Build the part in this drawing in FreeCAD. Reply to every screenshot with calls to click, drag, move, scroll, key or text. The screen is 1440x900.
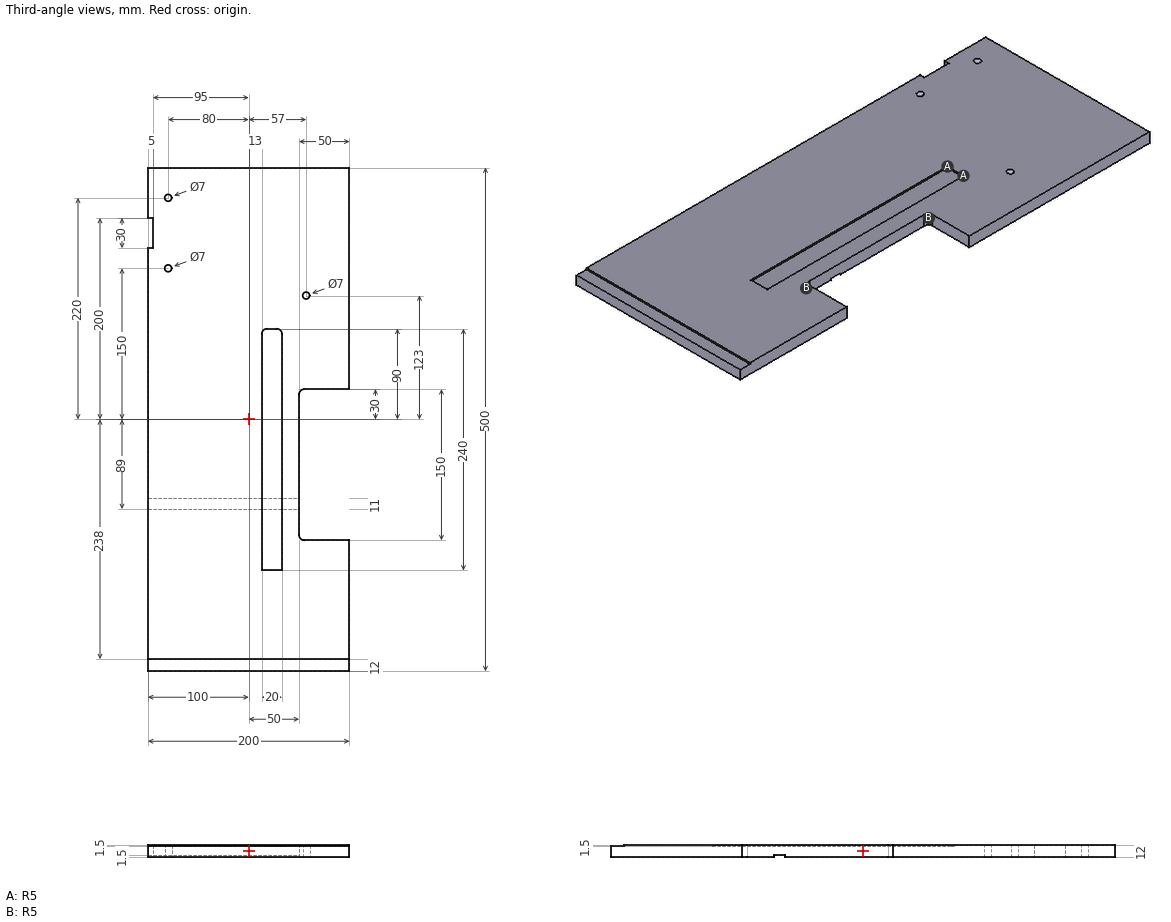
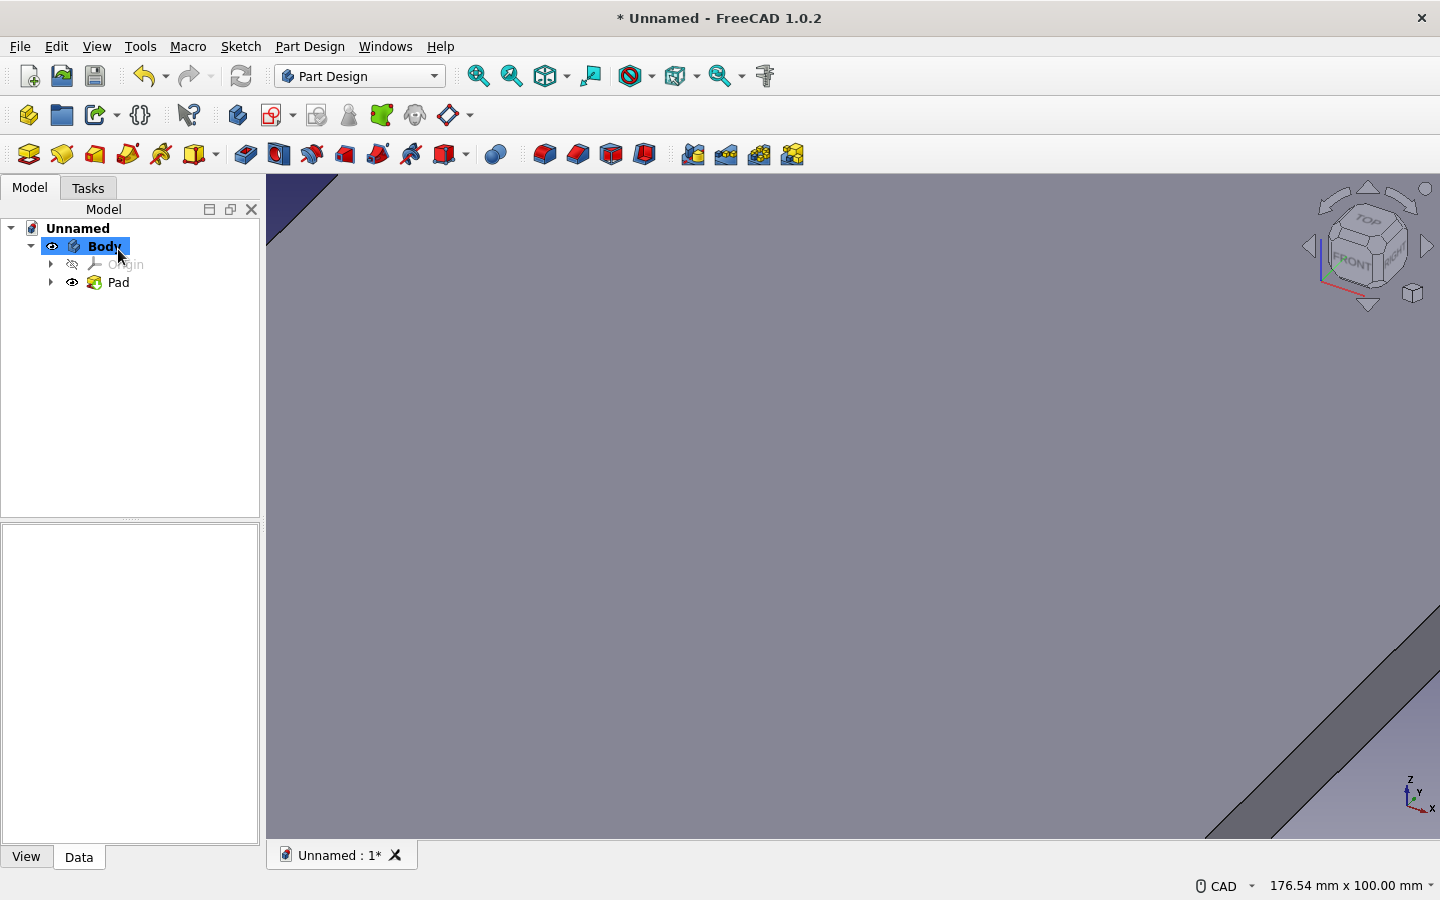
click(479, 76)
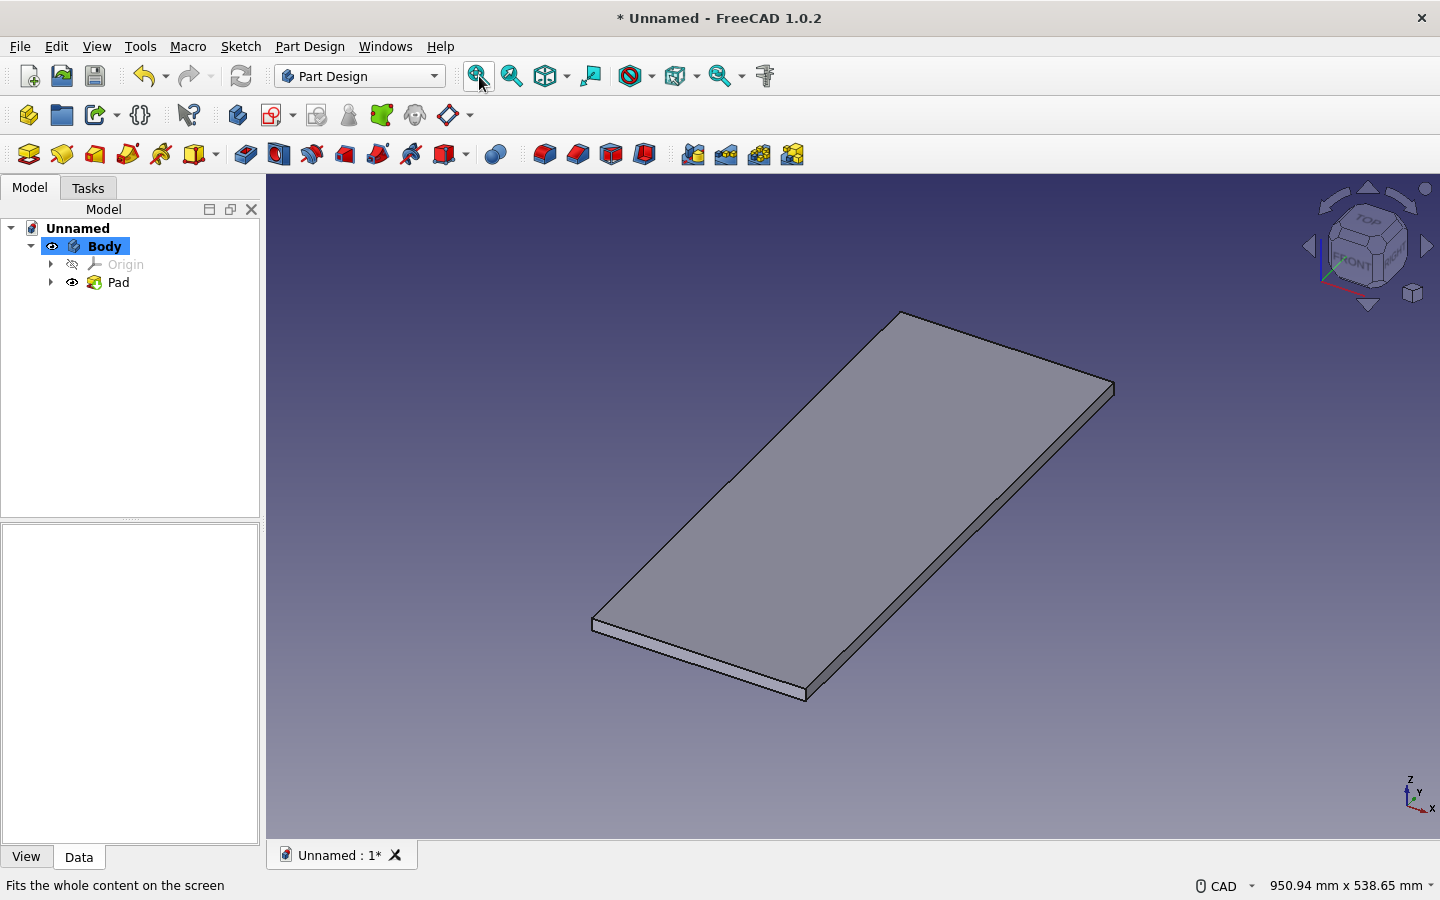
key(5)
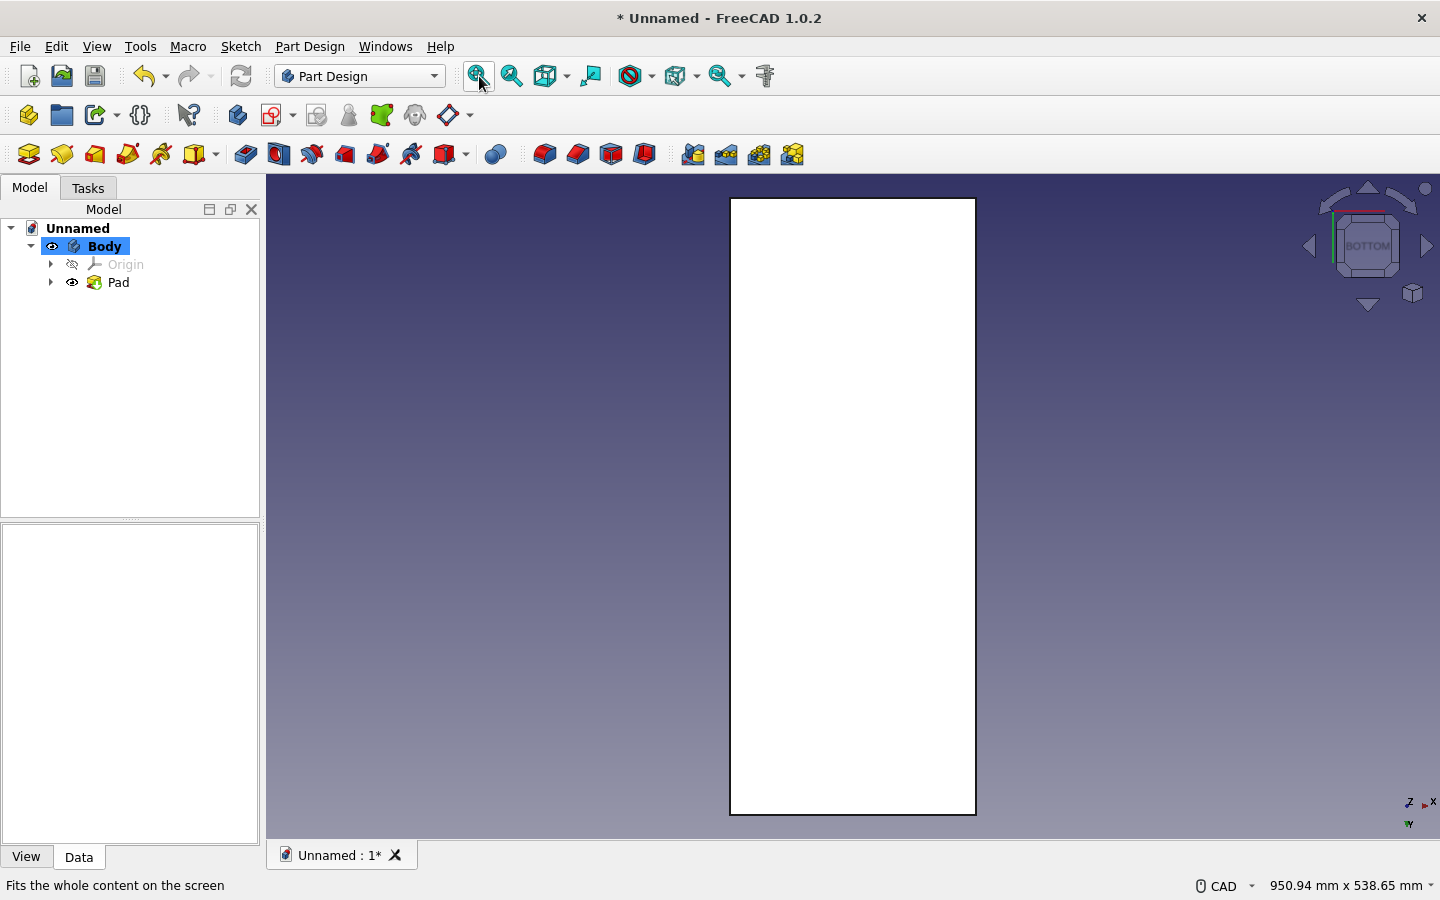
click(853, 682)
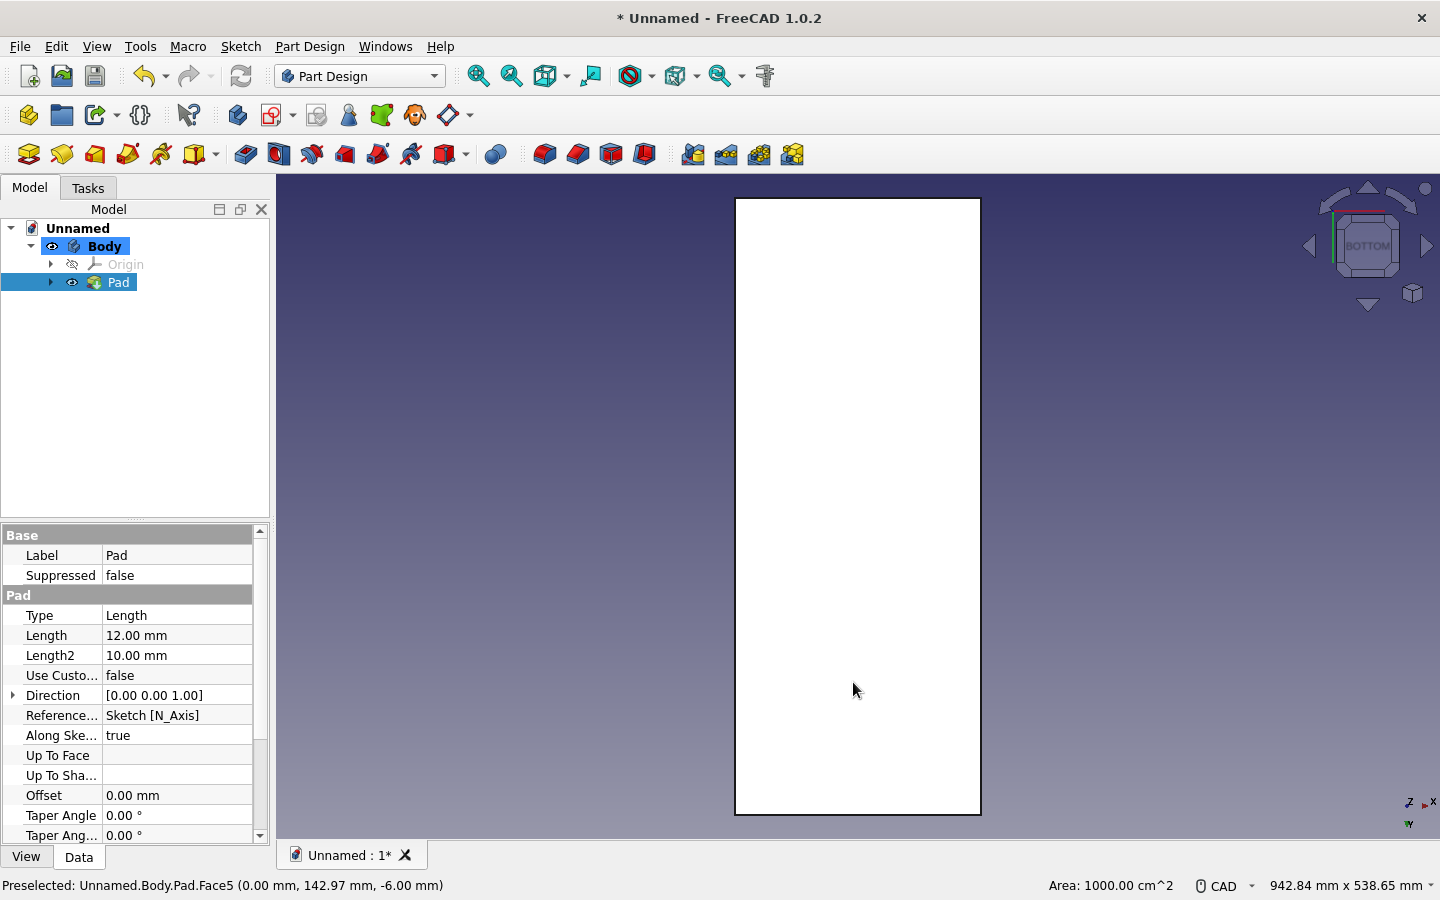
click(270, 116)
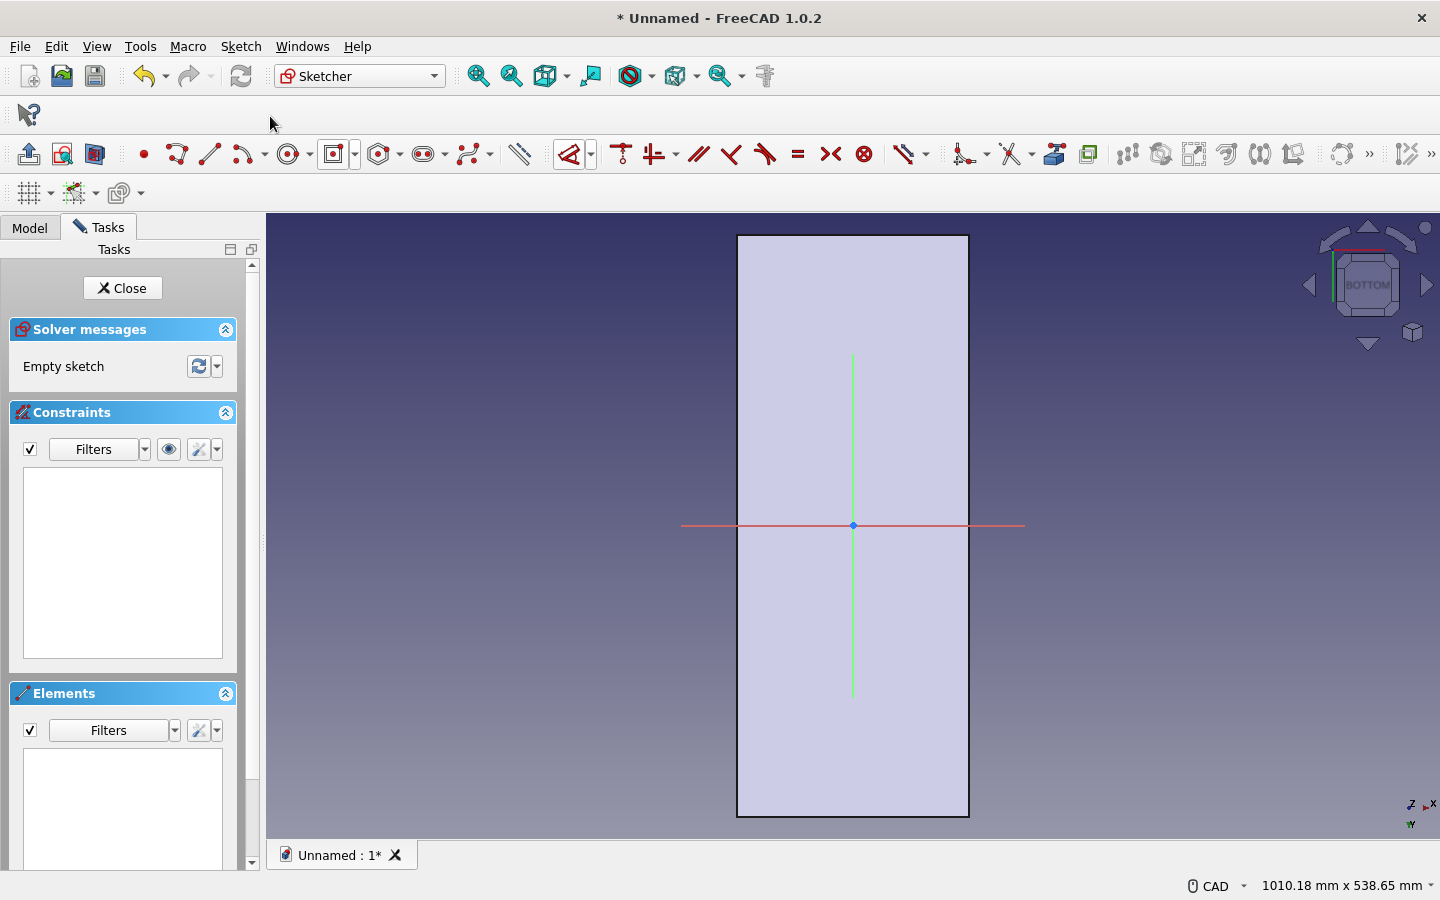
scroll(893, 444, up, 5)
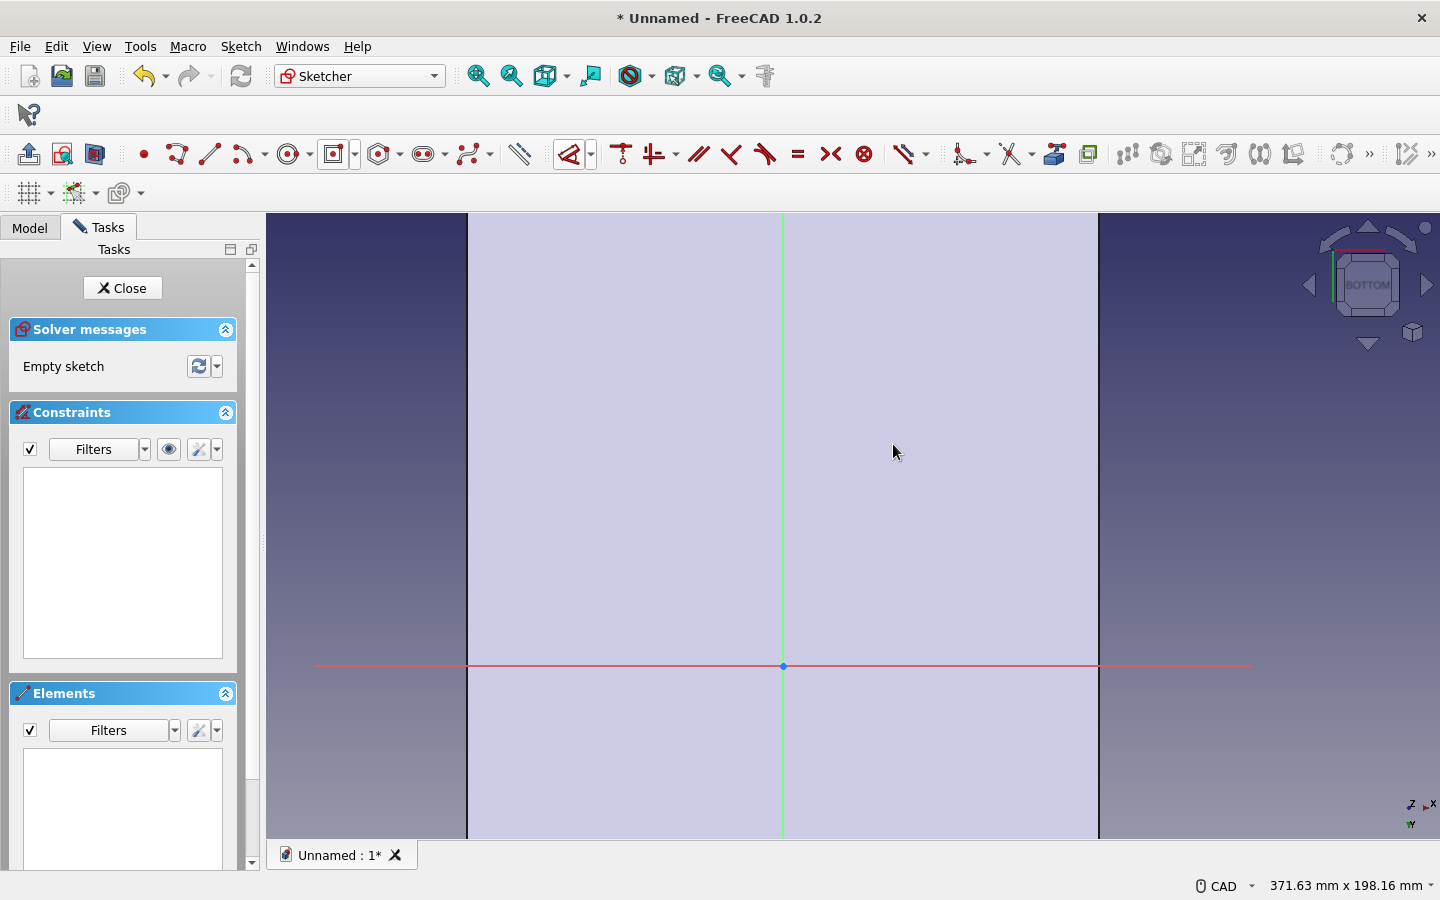
click(354, 154)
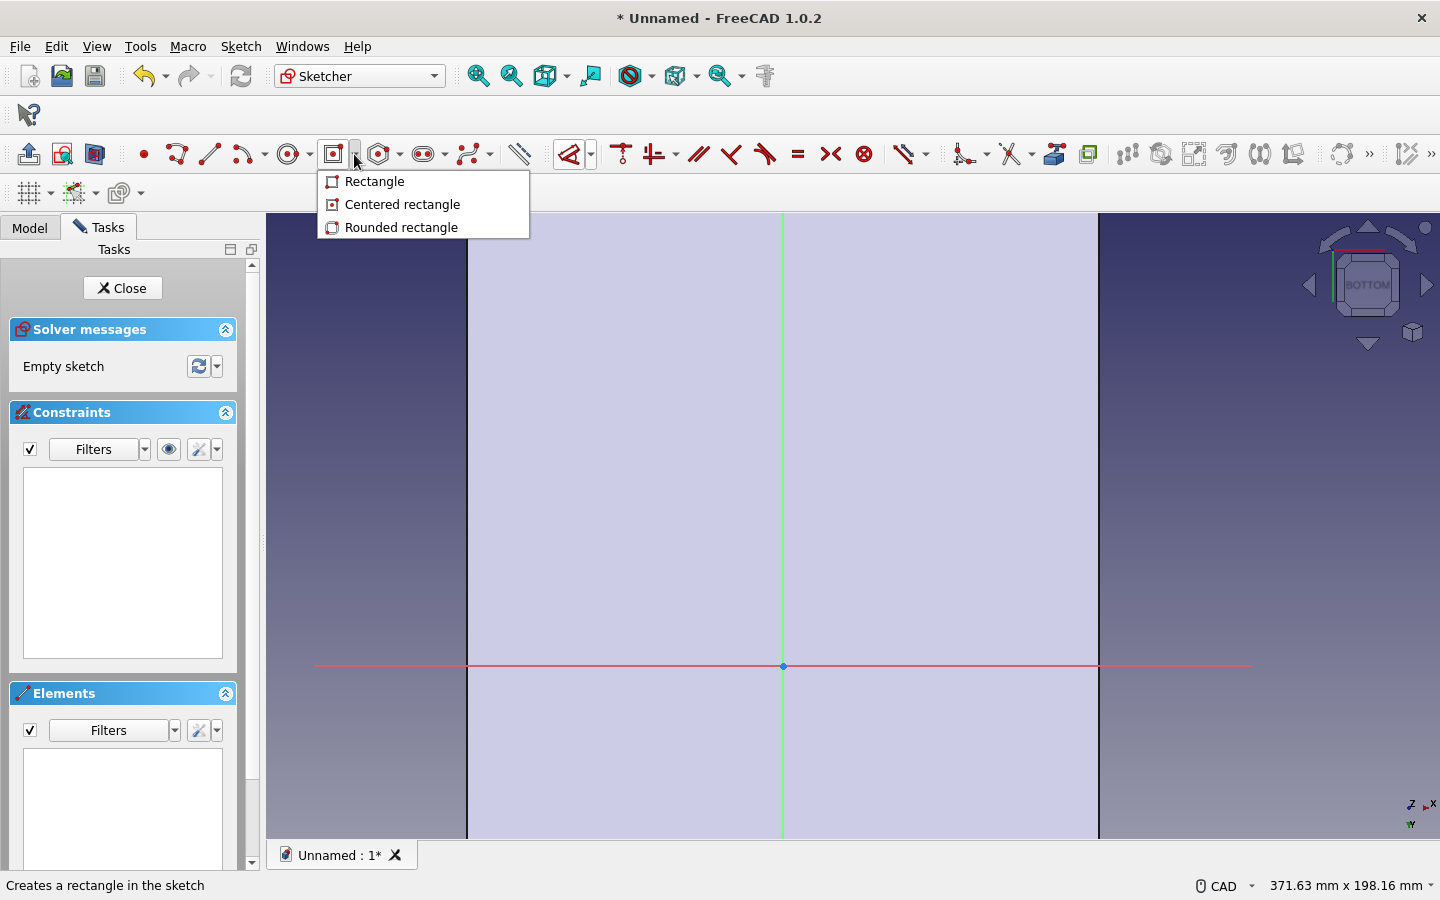
click(424, 182)